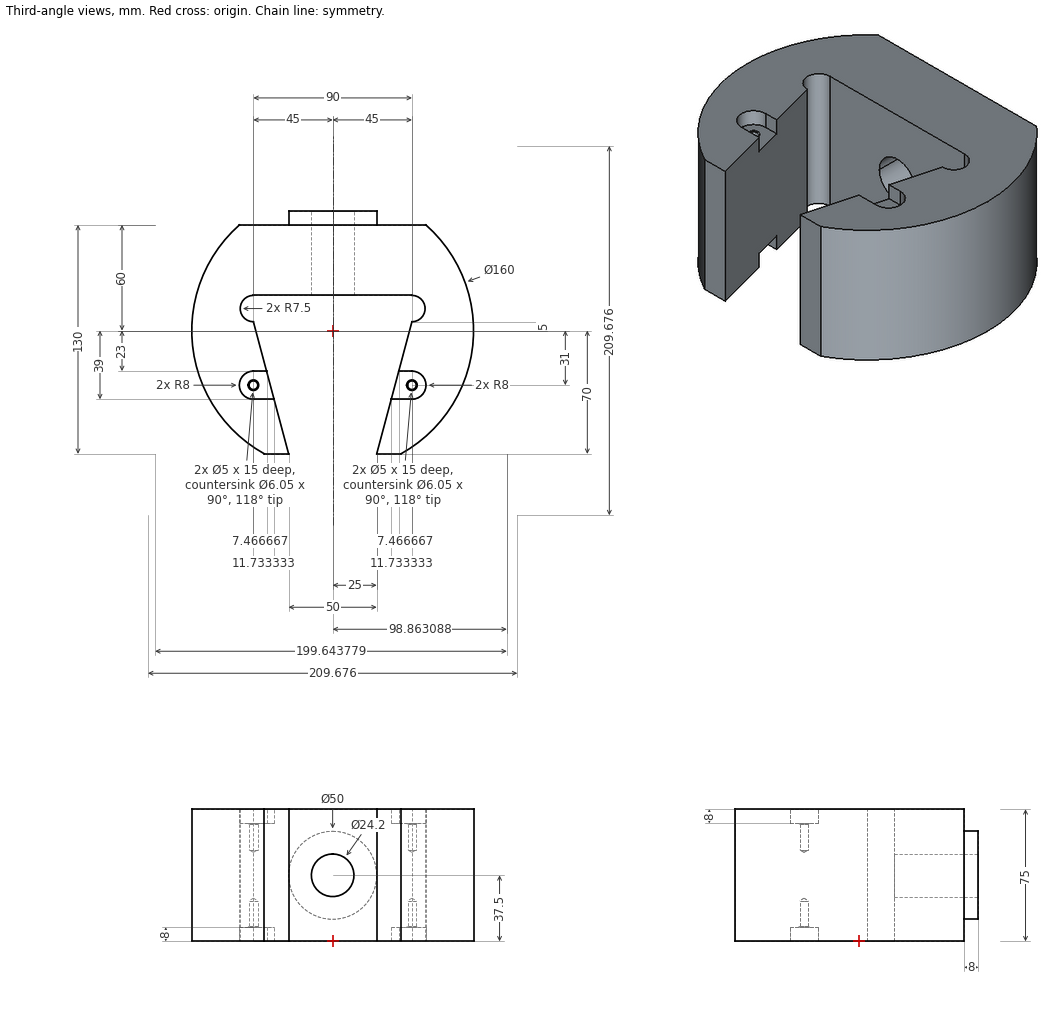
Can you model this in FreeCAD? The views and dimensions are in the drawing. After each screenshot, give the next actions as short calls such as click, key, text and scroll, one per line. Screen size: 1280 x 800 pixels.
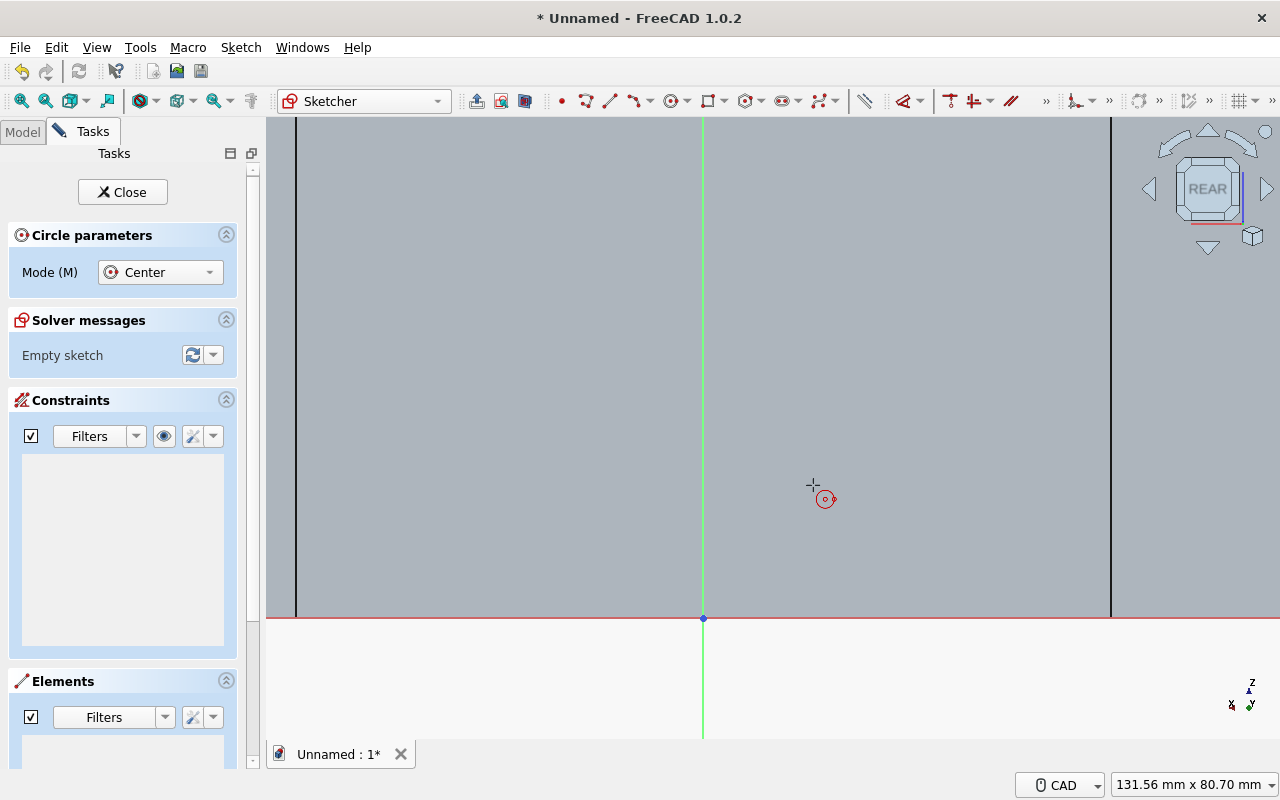
click(703, 329)
move(769, 263)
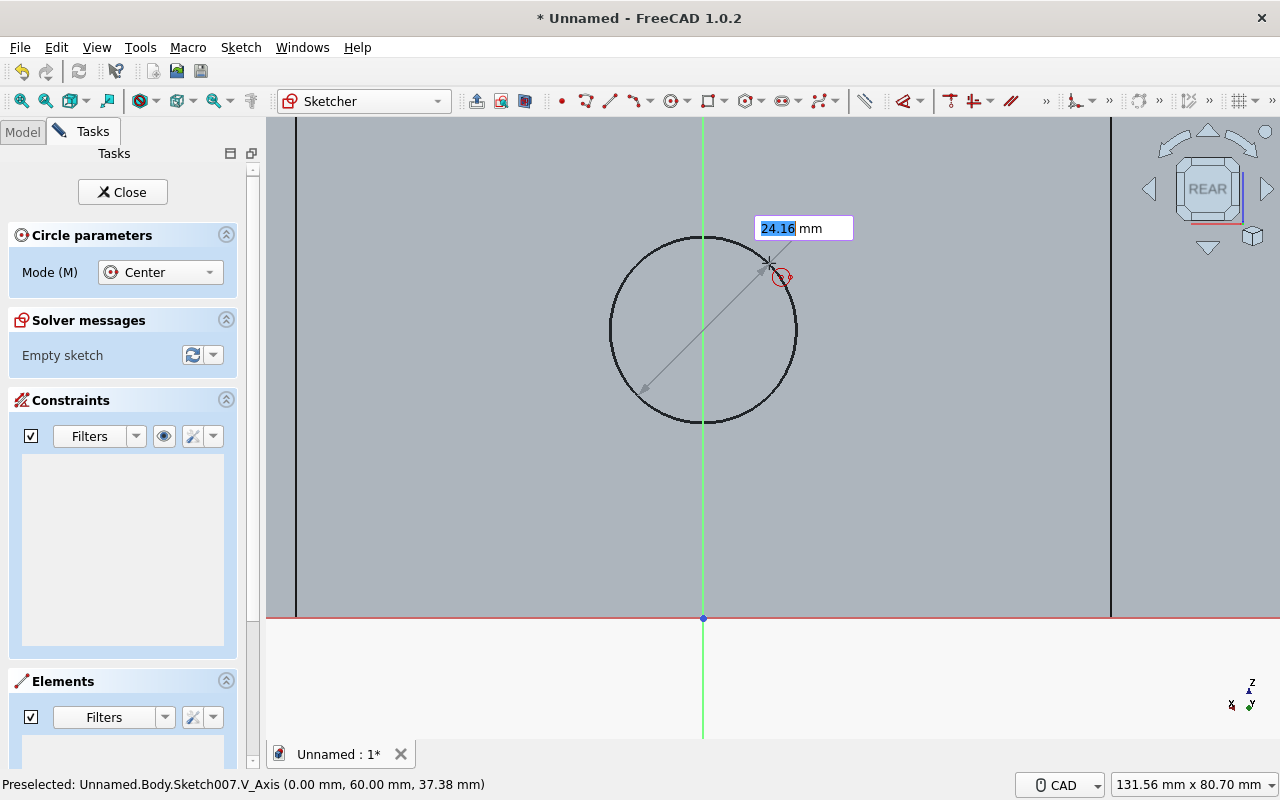
text(24.2)
key(Return)
key(Escape)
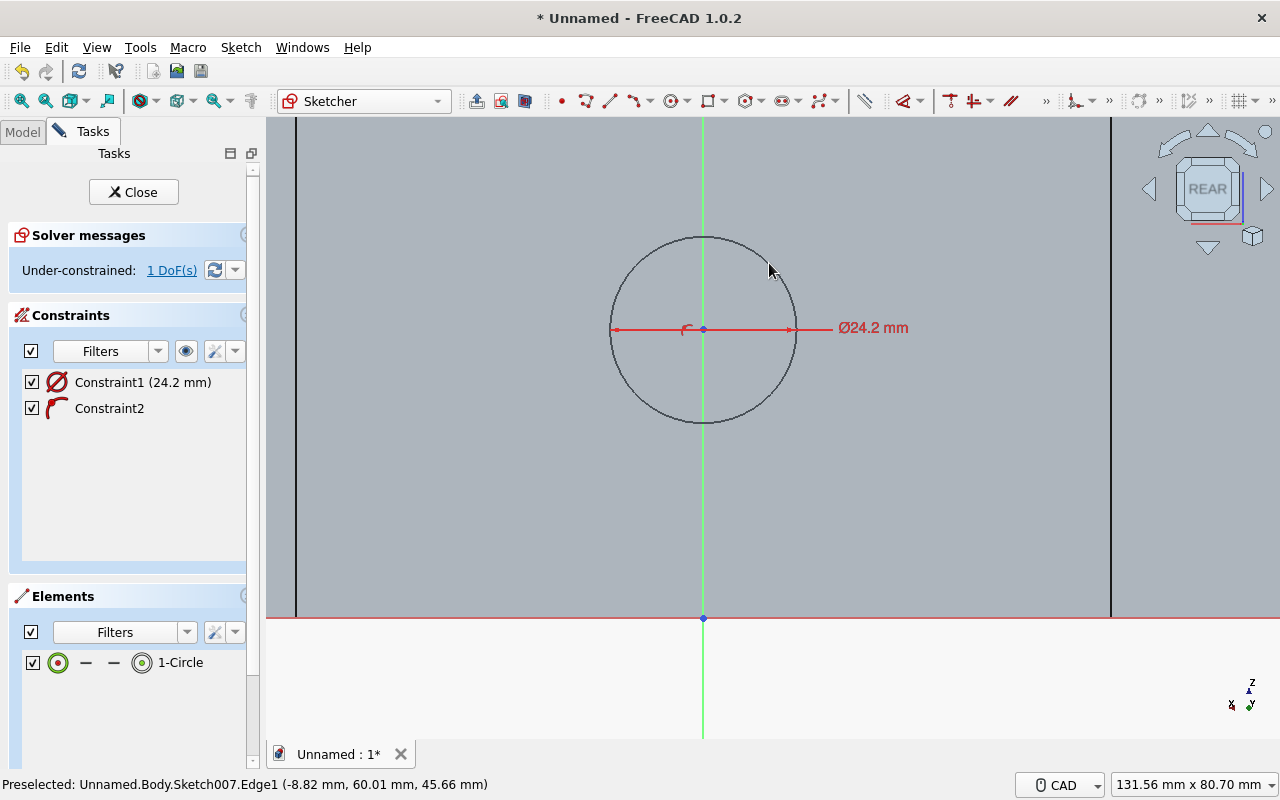
key(d)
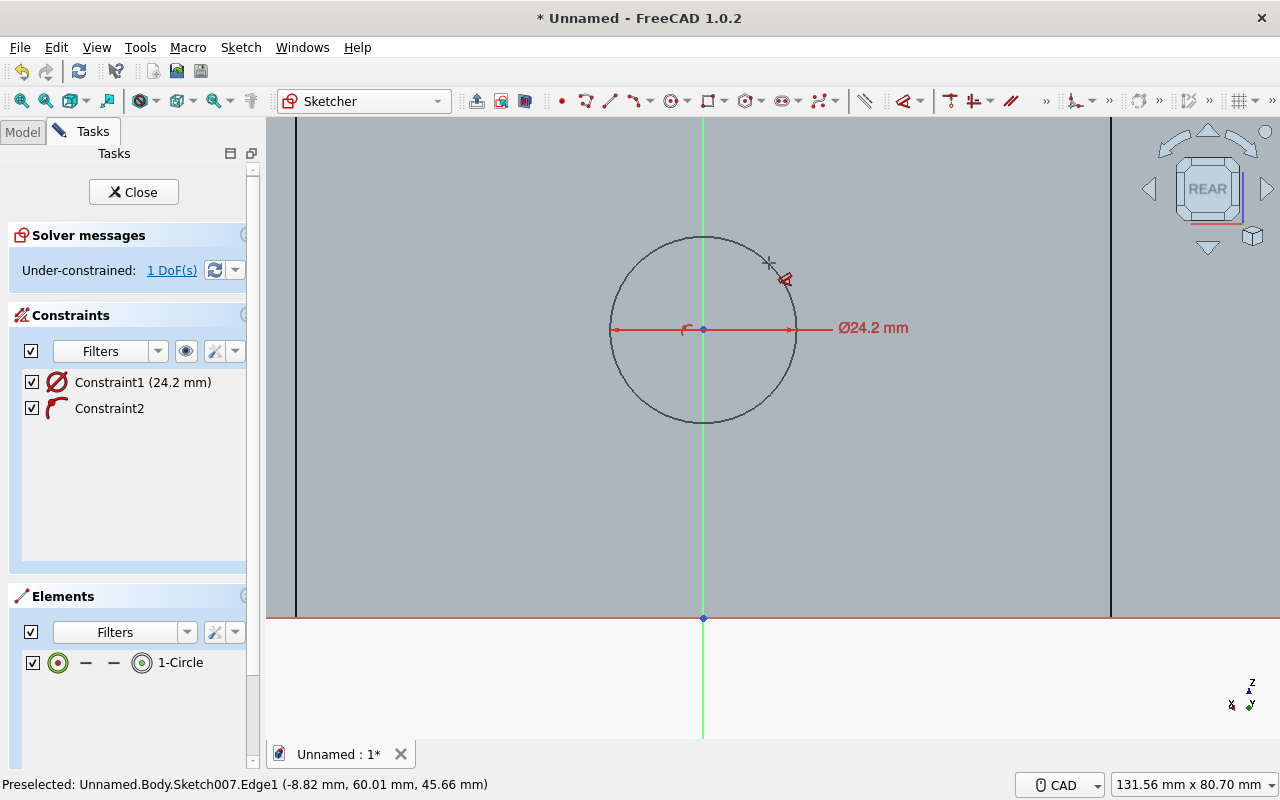
click(703, 330)
click(737, 474)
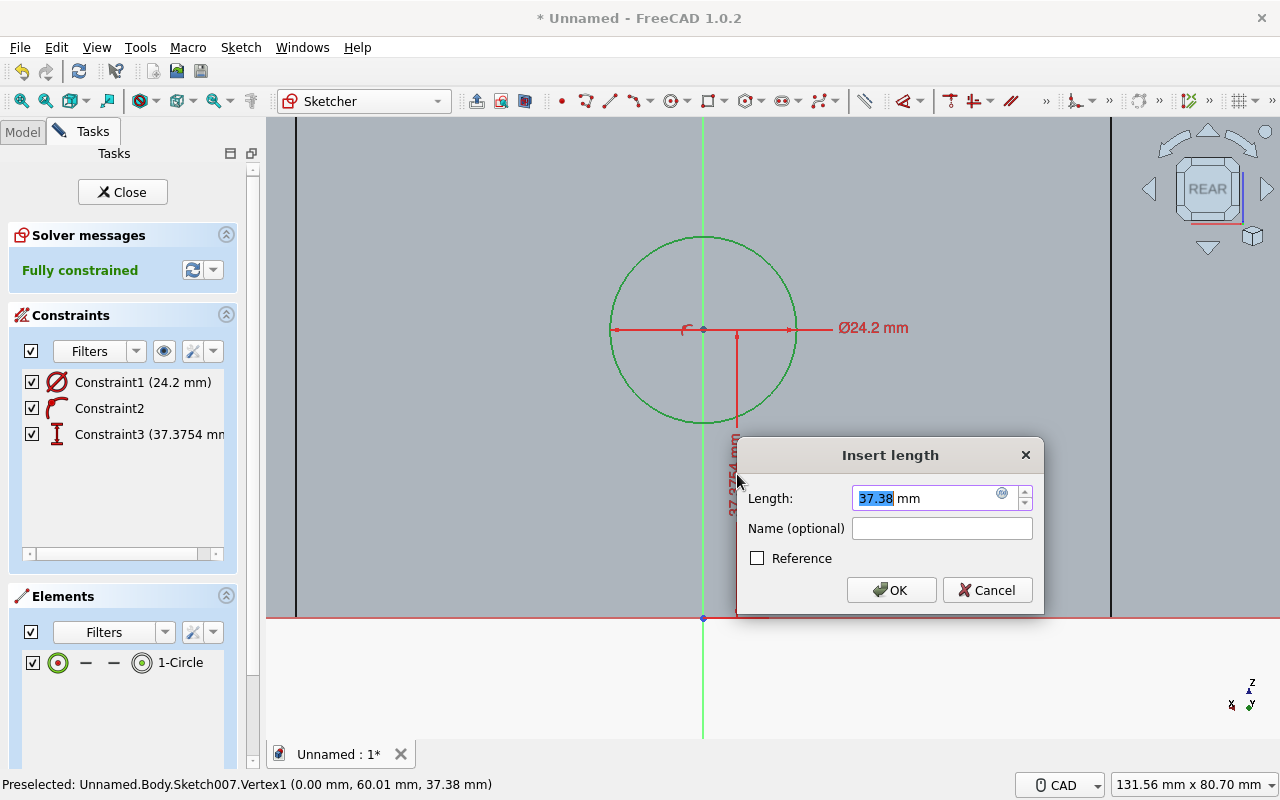
text(37.5)
key(Return)
key(Escape)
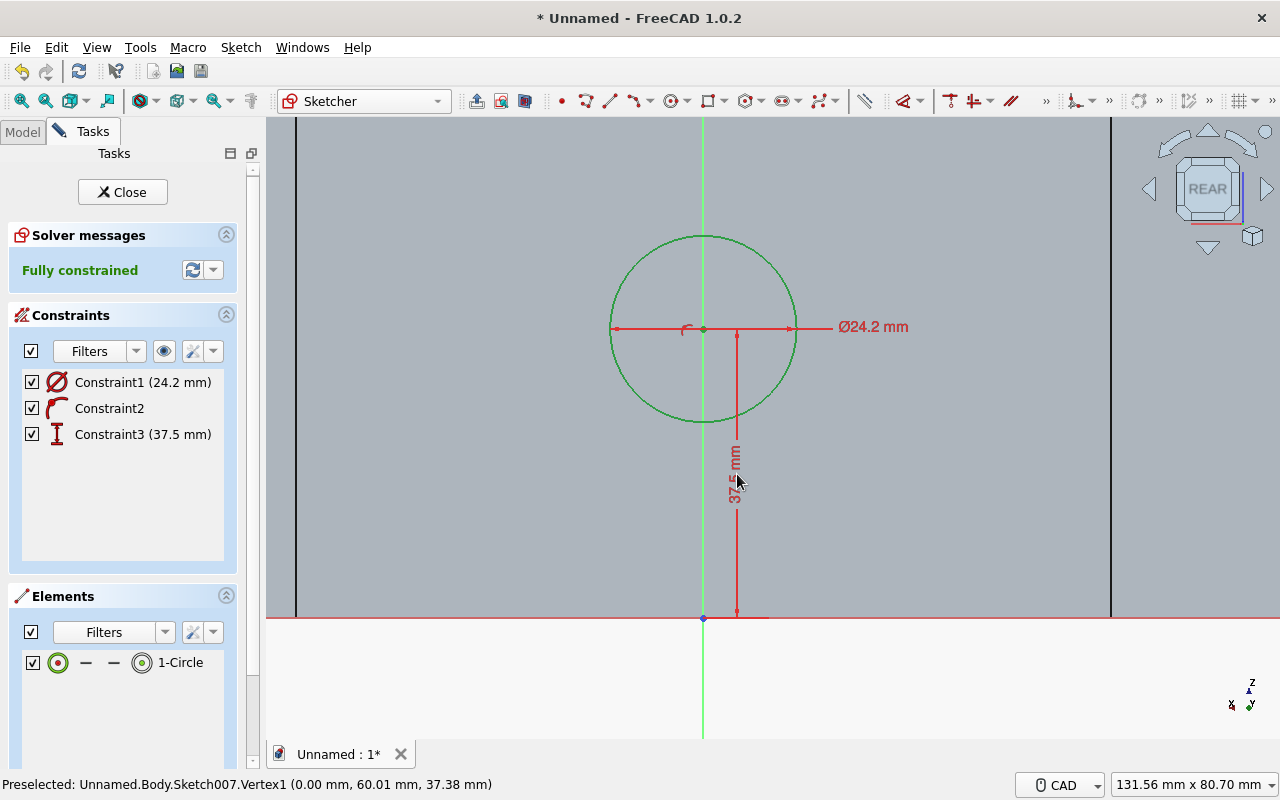
click(123, 192)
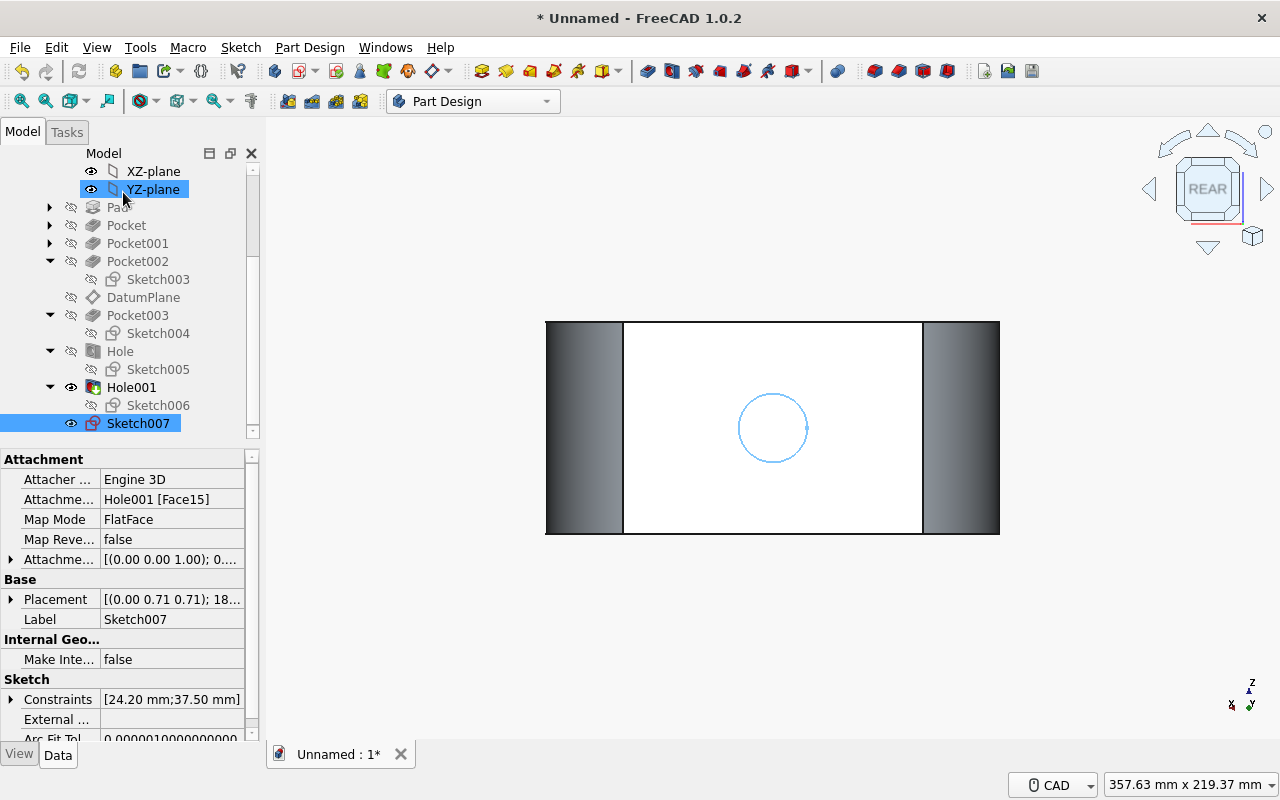
click(648, 72)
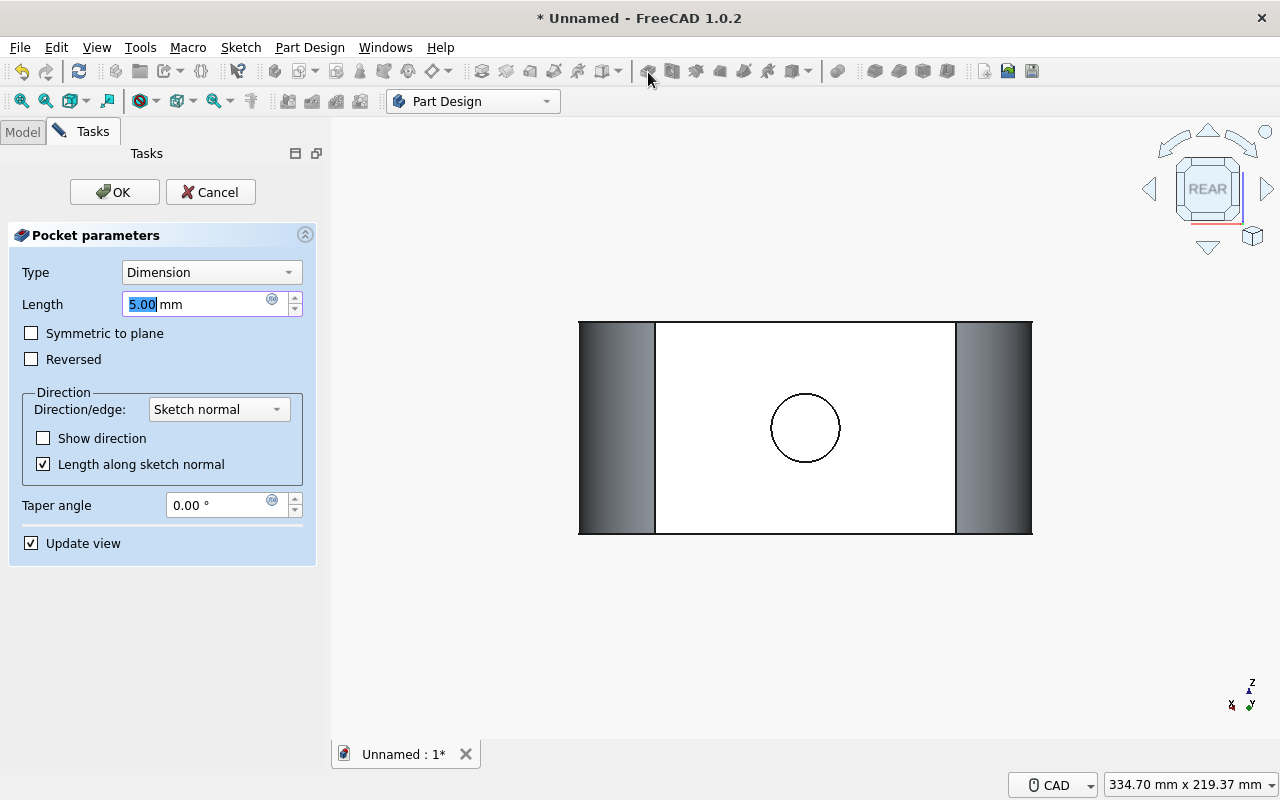
click(212, 272)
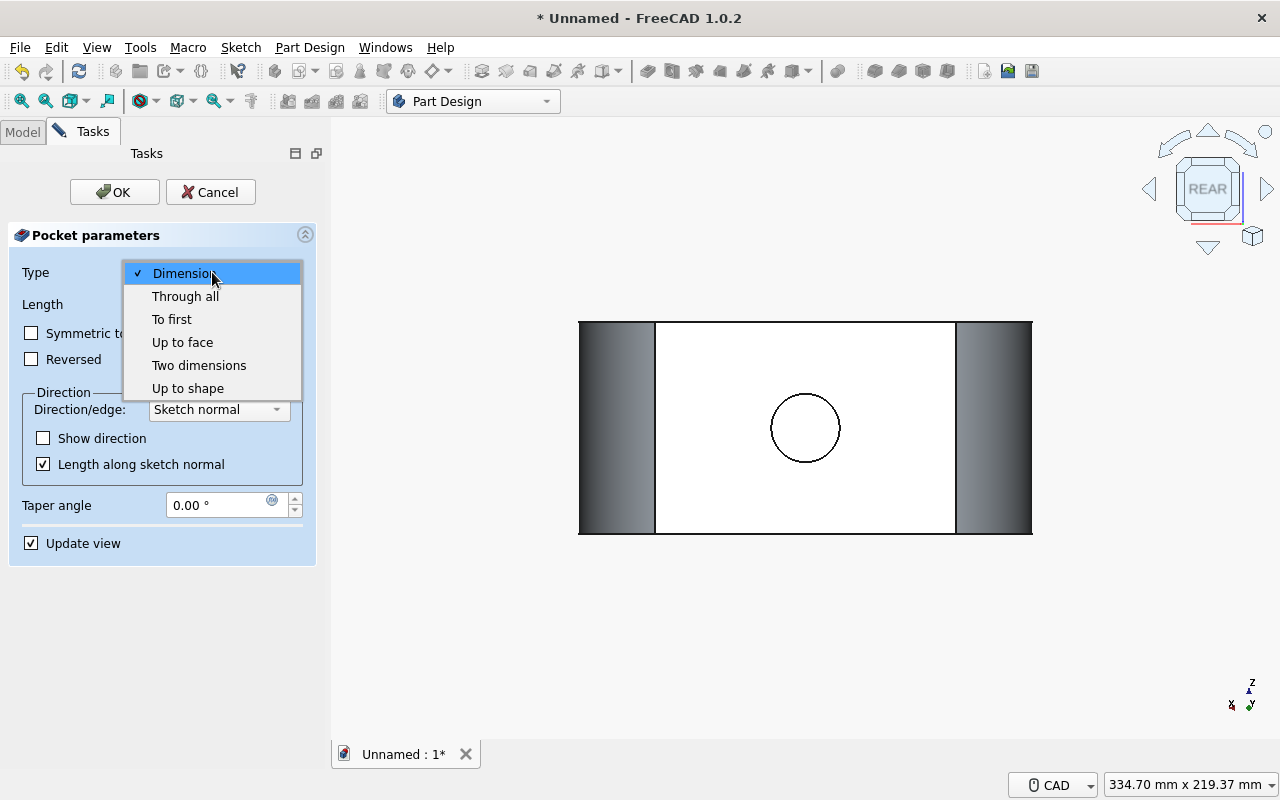
click(212, 320)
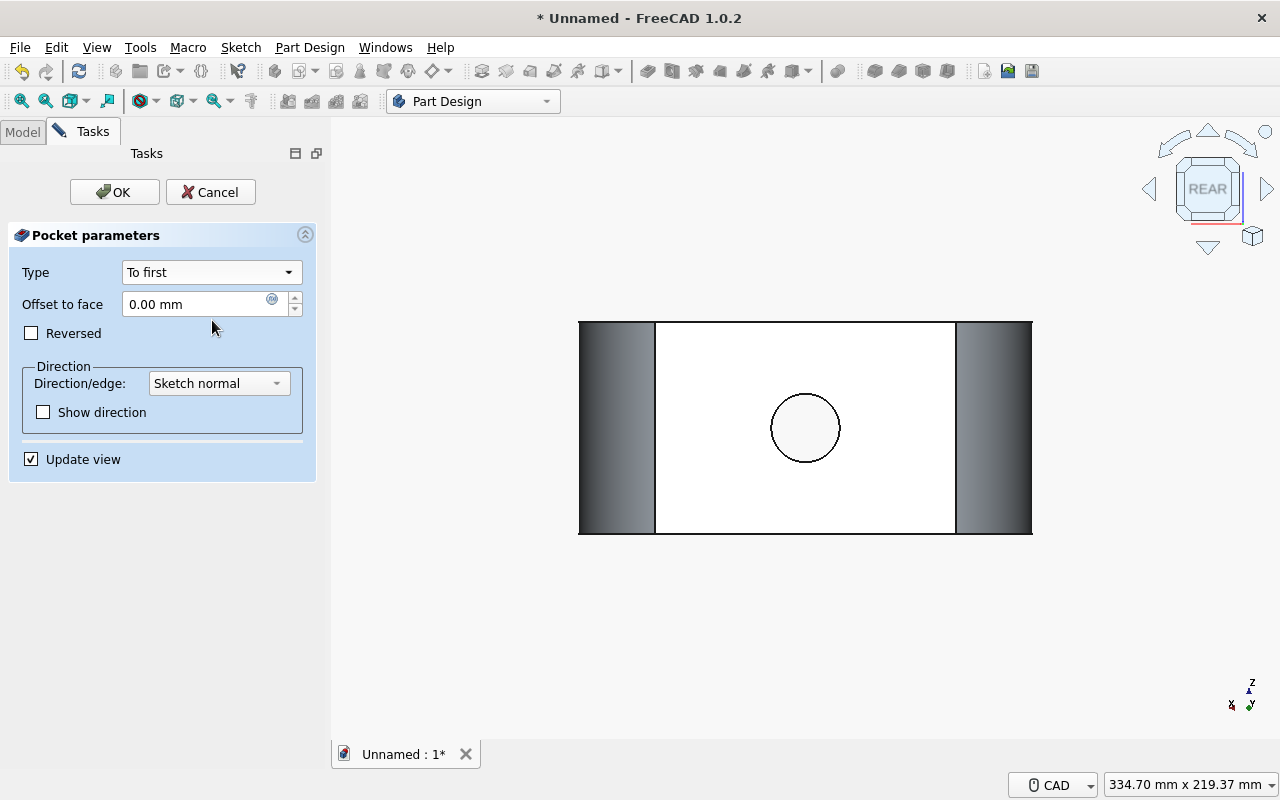
click(115, 192)